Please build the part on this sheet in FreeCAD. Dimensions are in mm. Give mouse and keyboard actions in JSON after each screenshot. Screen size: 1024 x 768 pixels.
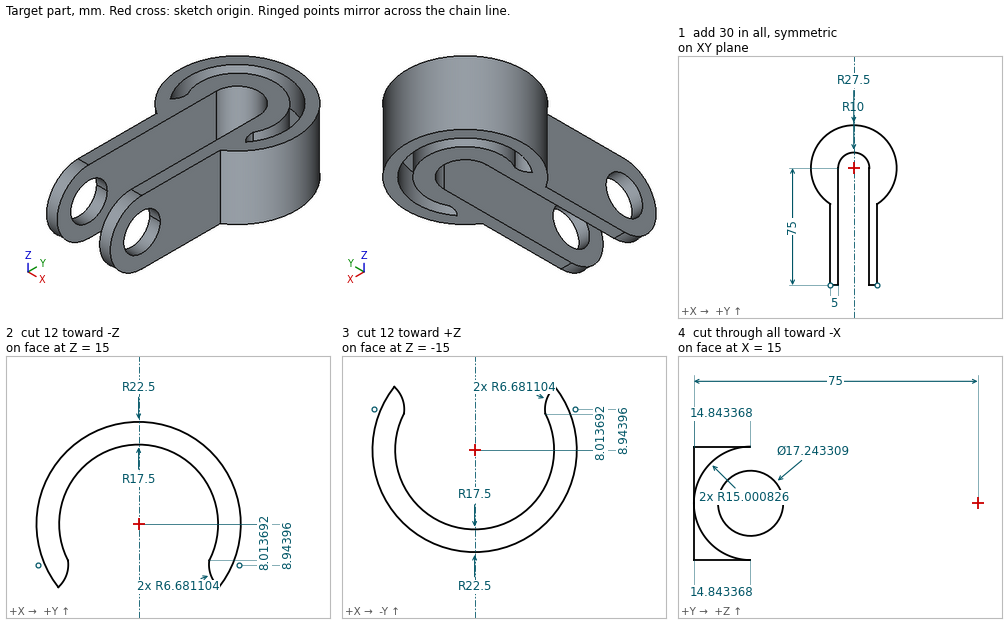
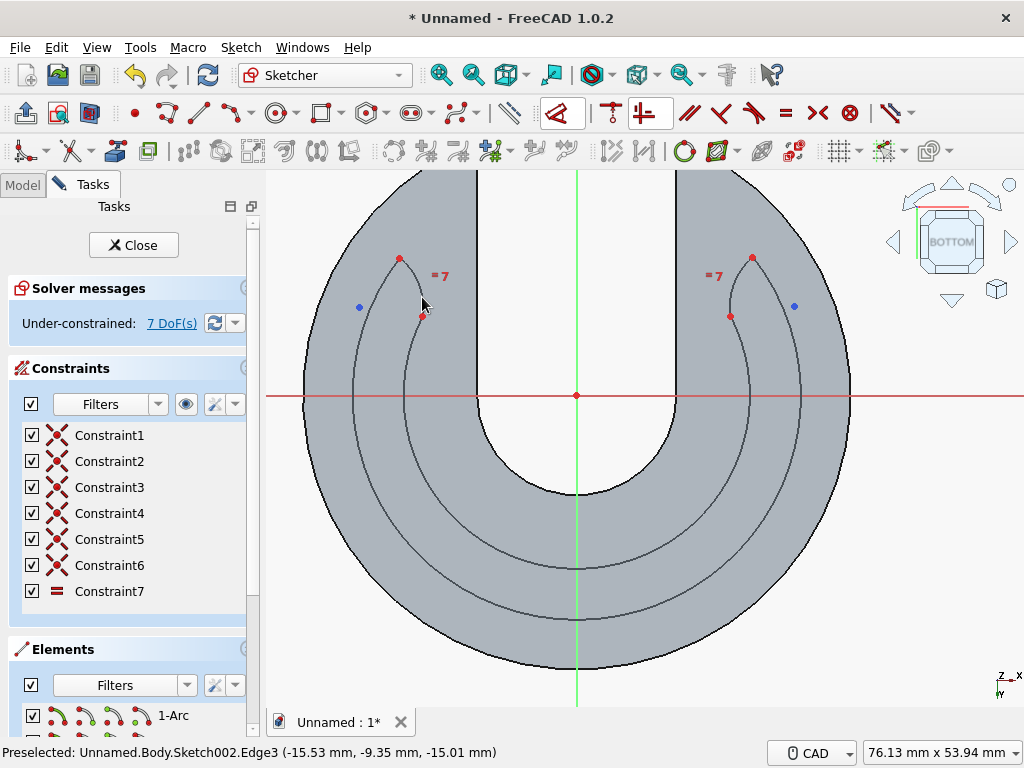
{"action": "left_click", "coordinate": [794, 306]}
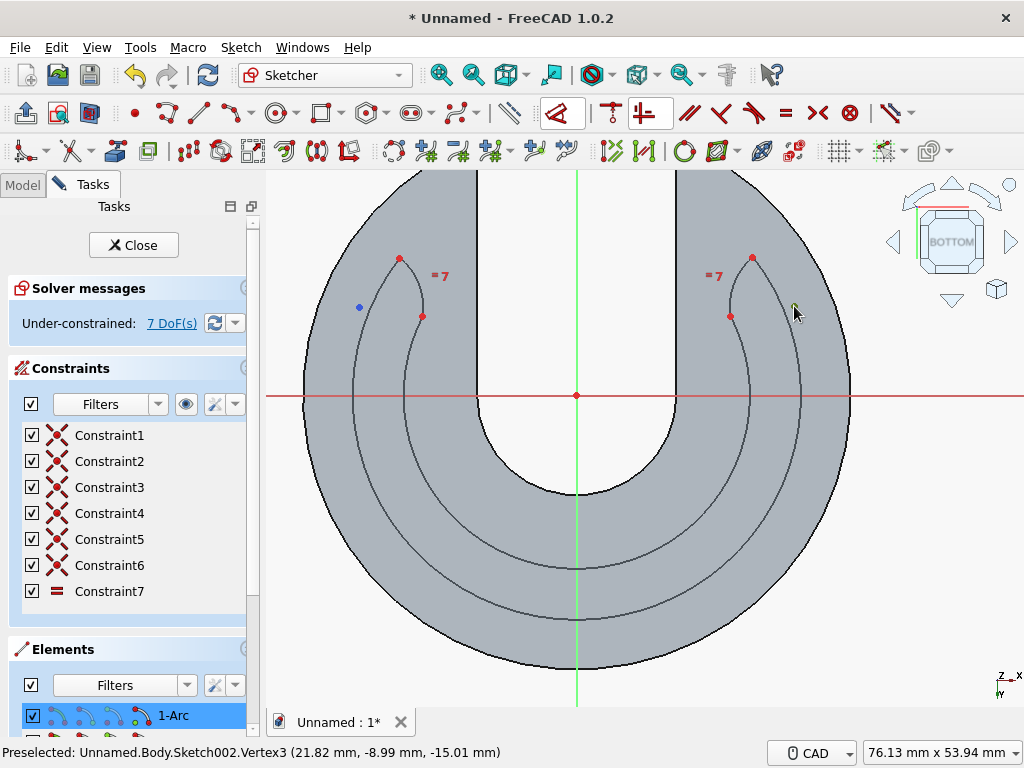
{"action": "left_click", "coordinate": [359, 307]}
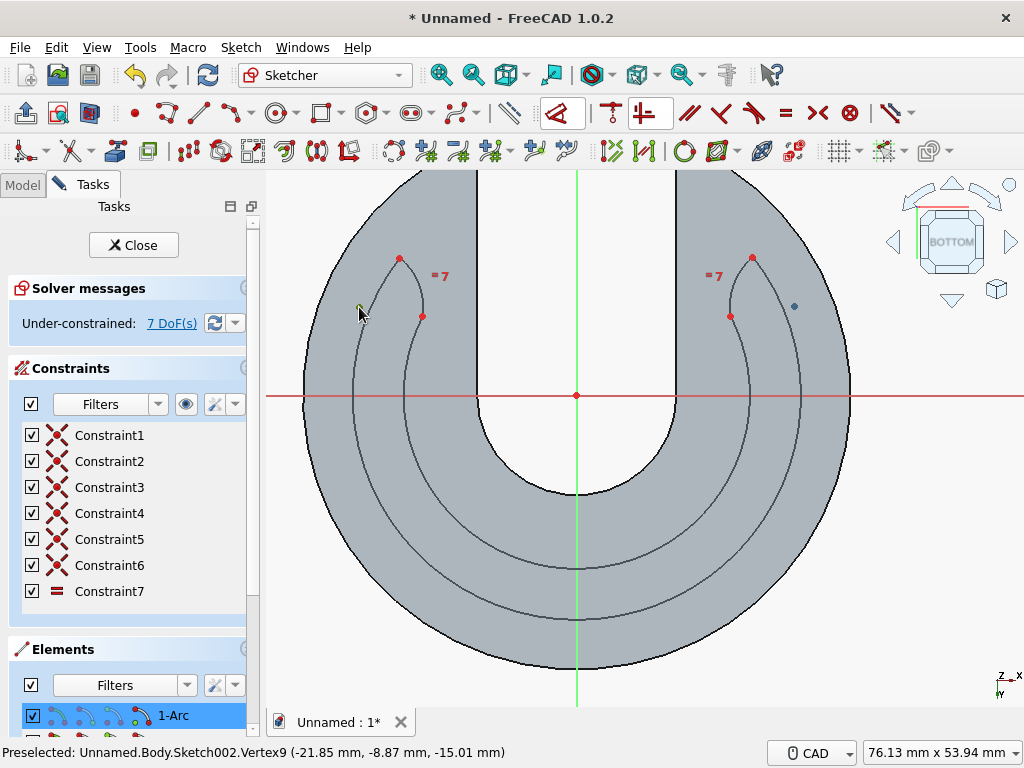
{"action": "left_click", "coordinate": [577, 507]}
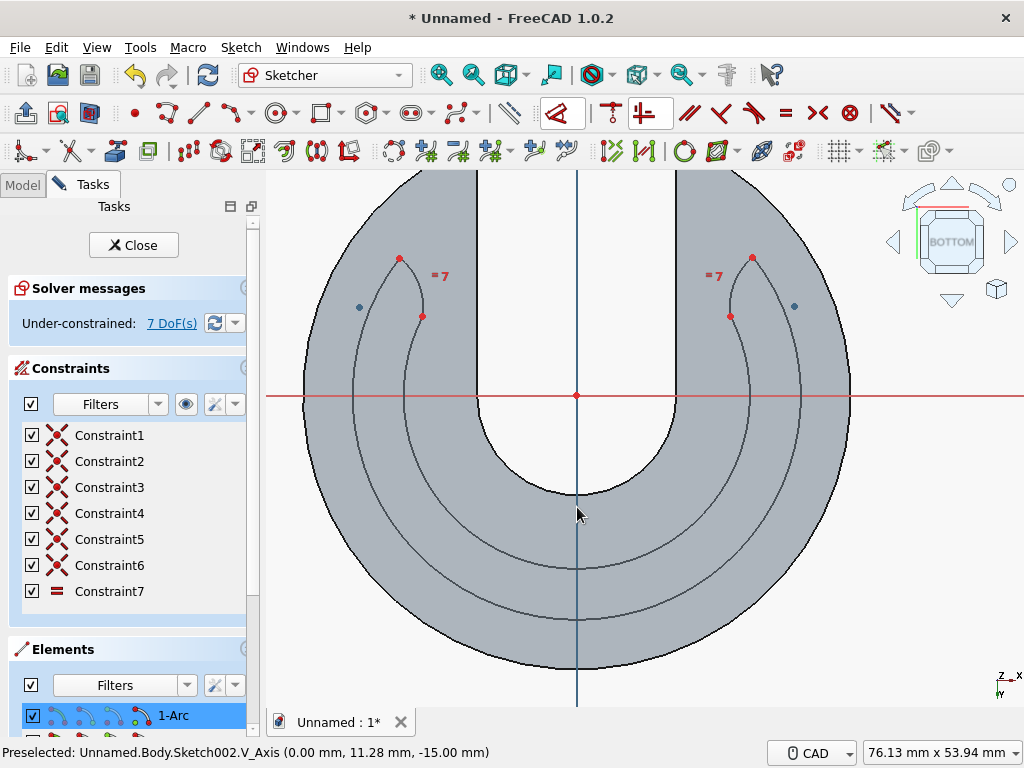
{"action": "left_click", "coordinate": [818, 114]}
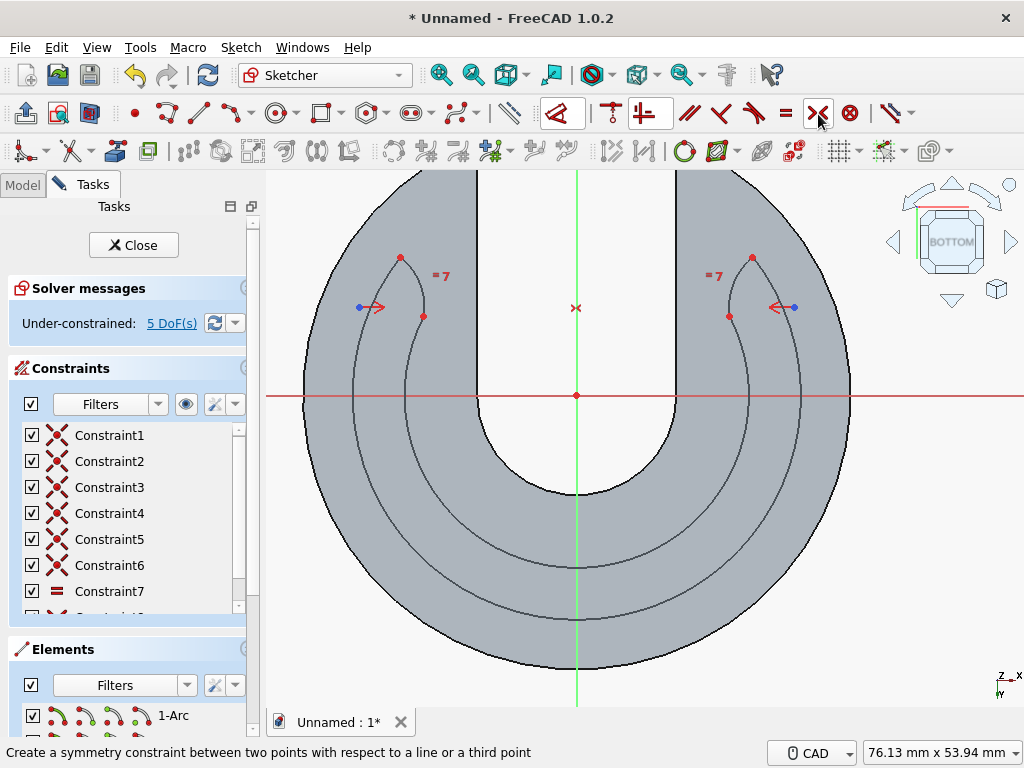
{"action": "left_click", "coordinate": [740, 272]}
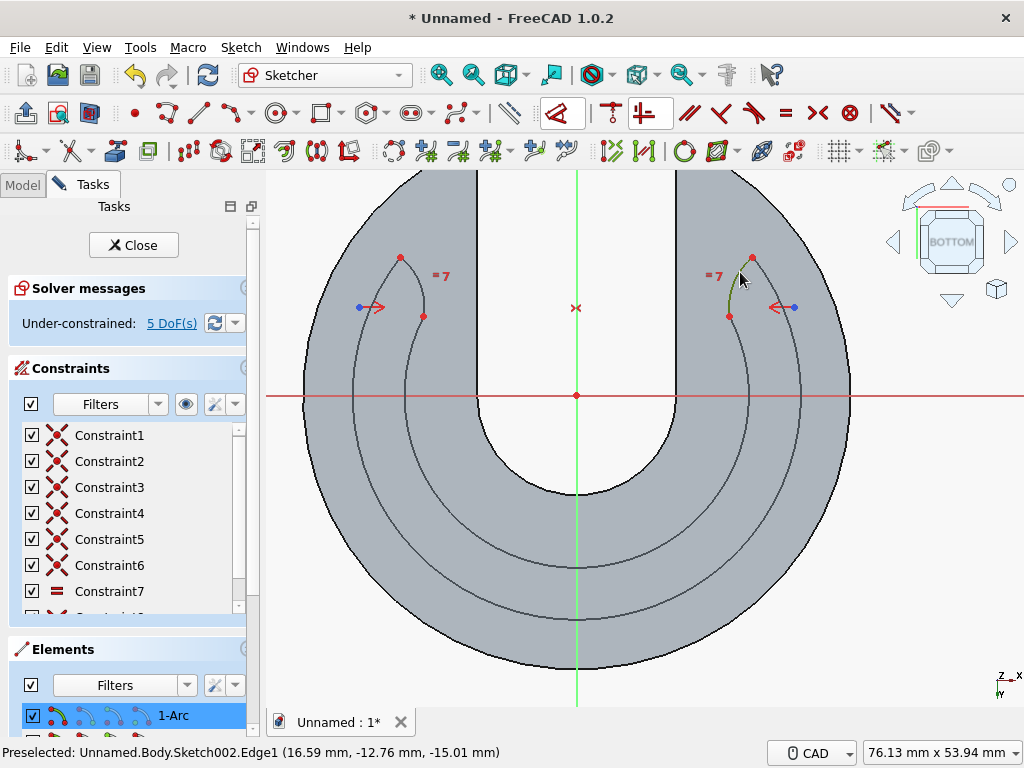
{"action": "key", "text": "k r"}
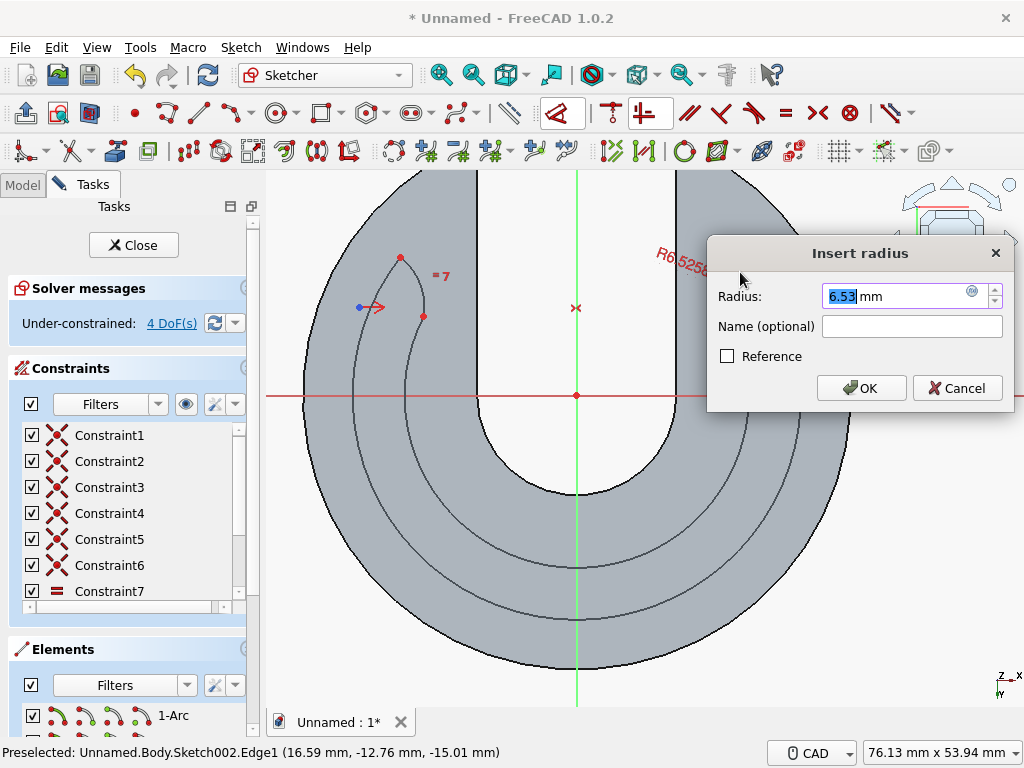
{"action": "type", "text": "6.681104"}
{"action": "key", "text": "Return"}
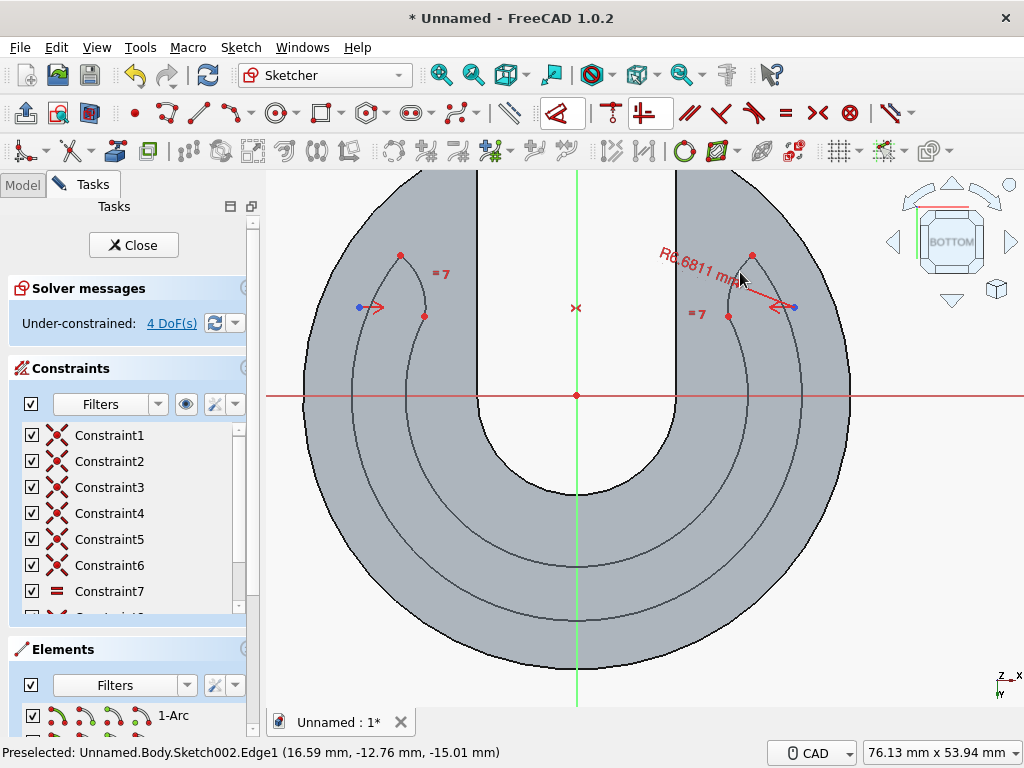
{"action": "left_click", "coordinate": [401, 536]}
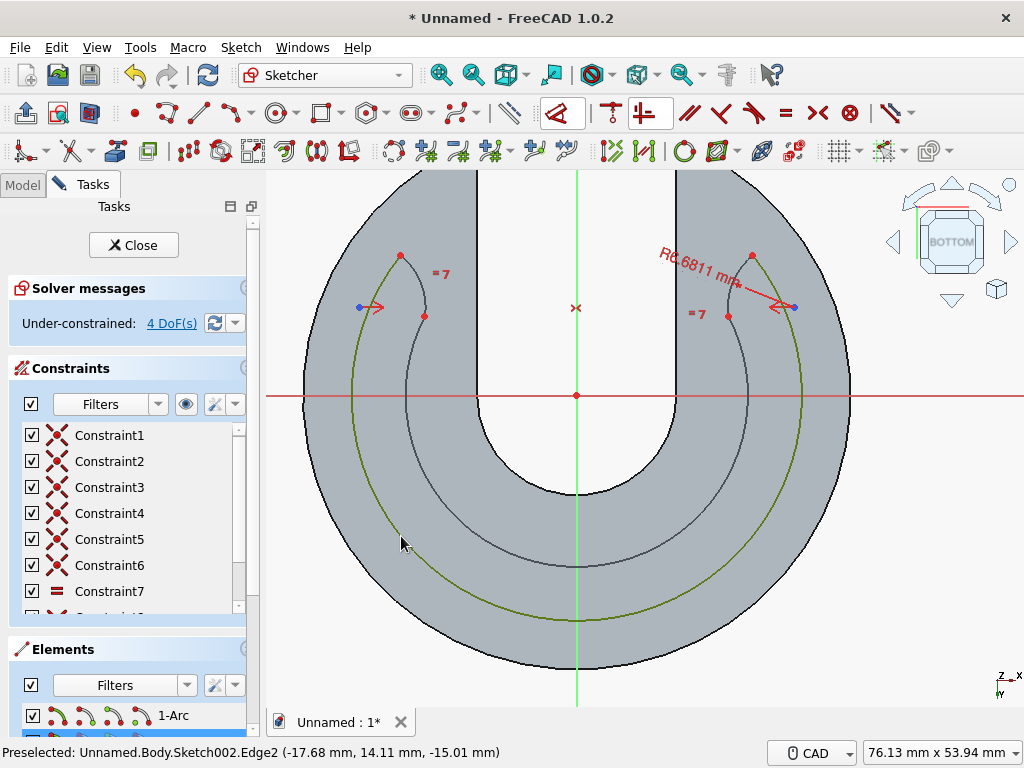
{"action": "key", "text": "k r"}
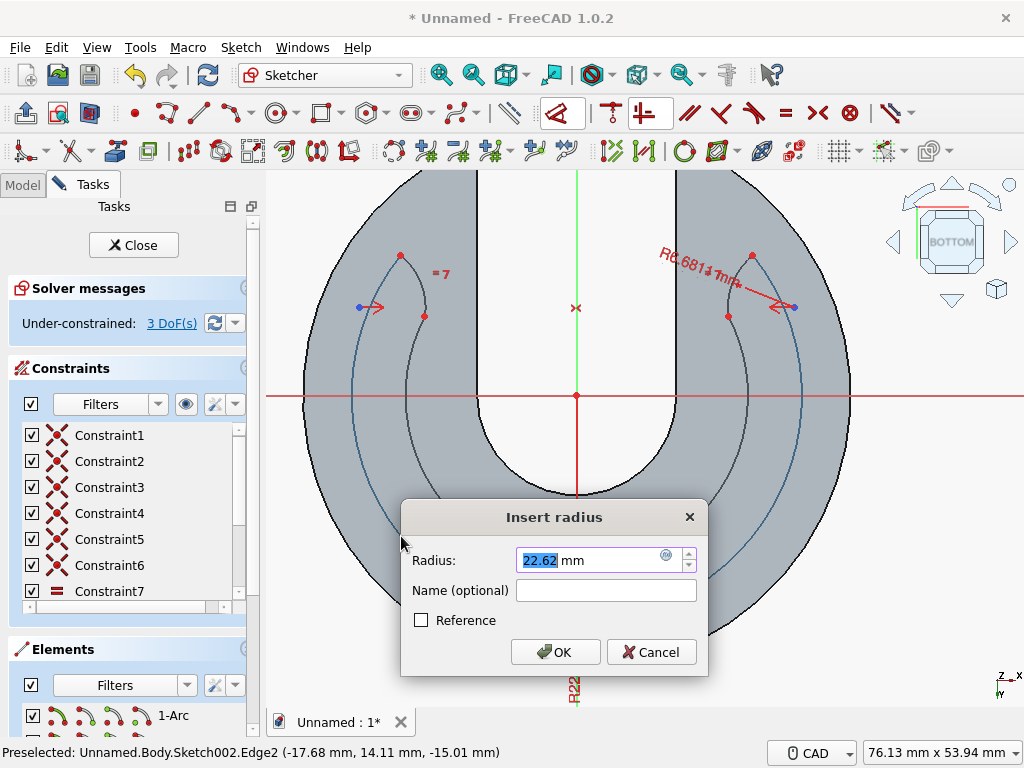
{"action": "type", "text": "22.5"}
{"action": "key", "text": "Return"}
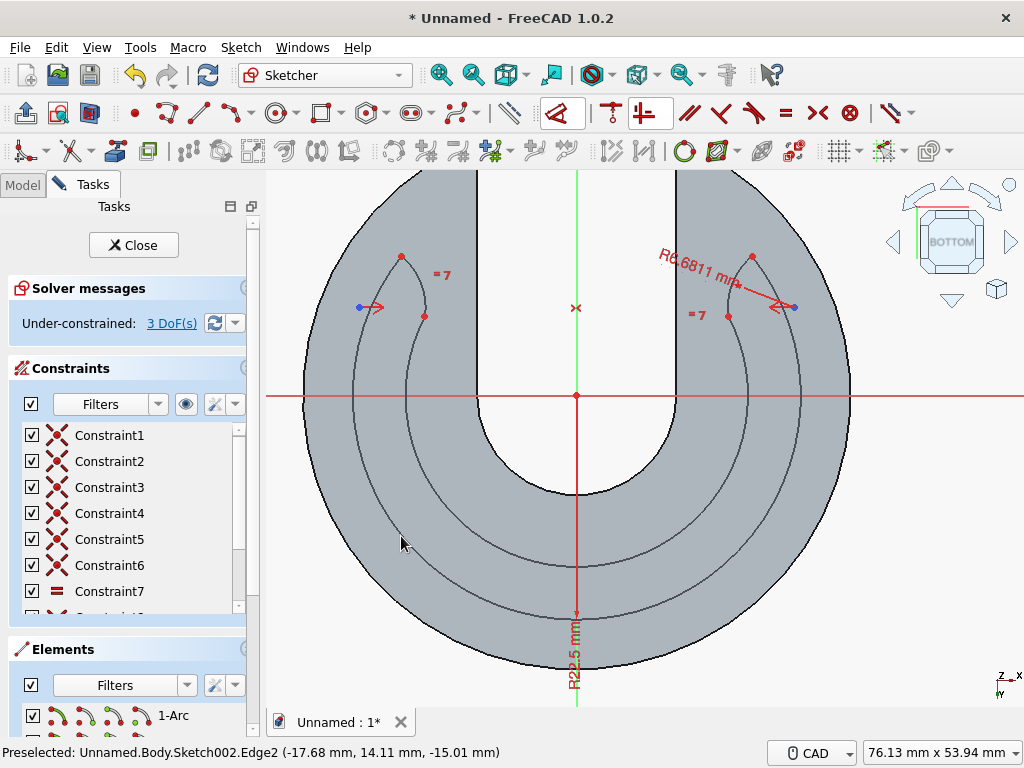
{"action": "left_click", "coordinate": [452, 513]}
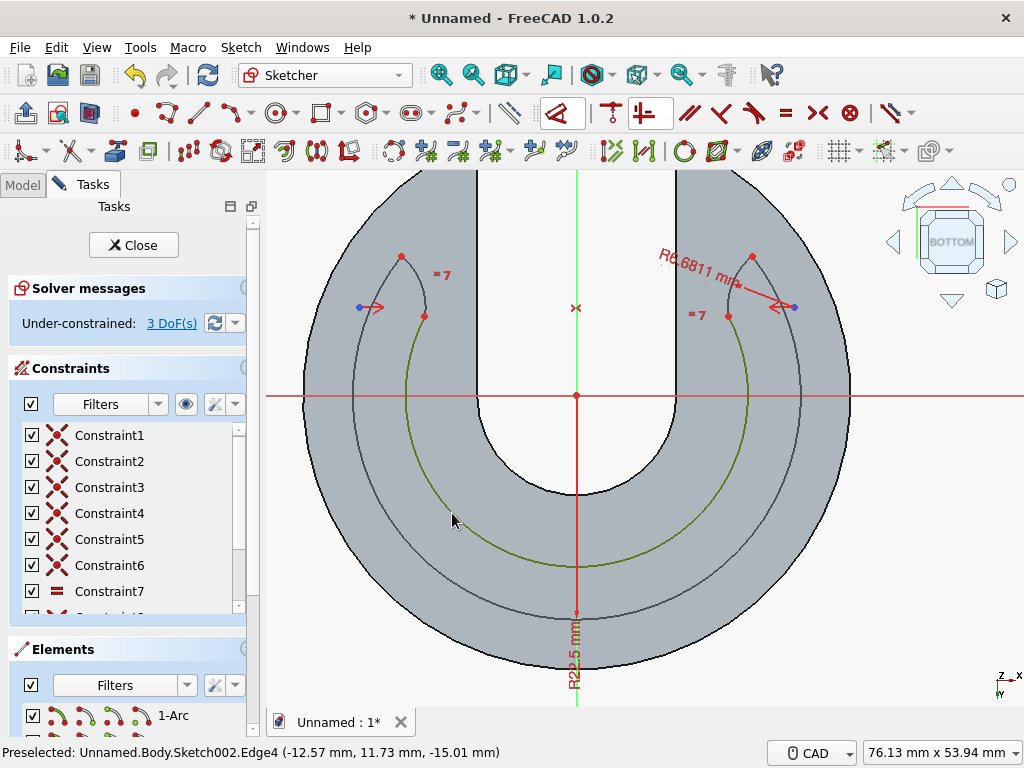
{"action": "key", "text": "k r"}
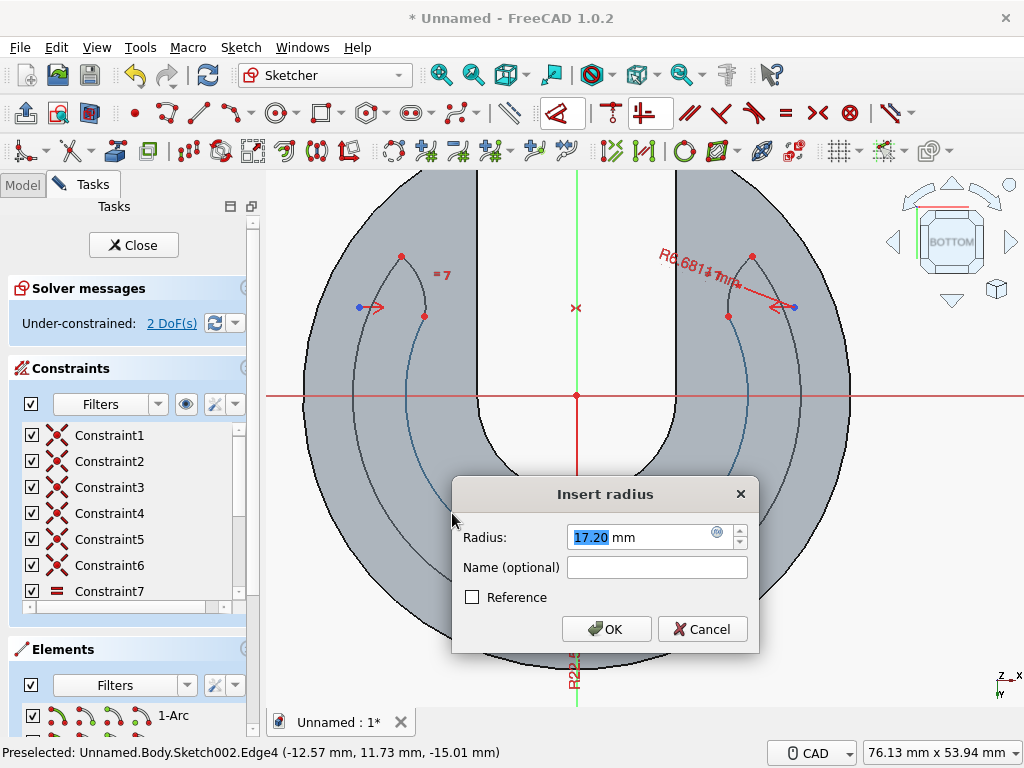
{"action": "type", "text": "17.5"}
{"action": "key", "text": "Return"}